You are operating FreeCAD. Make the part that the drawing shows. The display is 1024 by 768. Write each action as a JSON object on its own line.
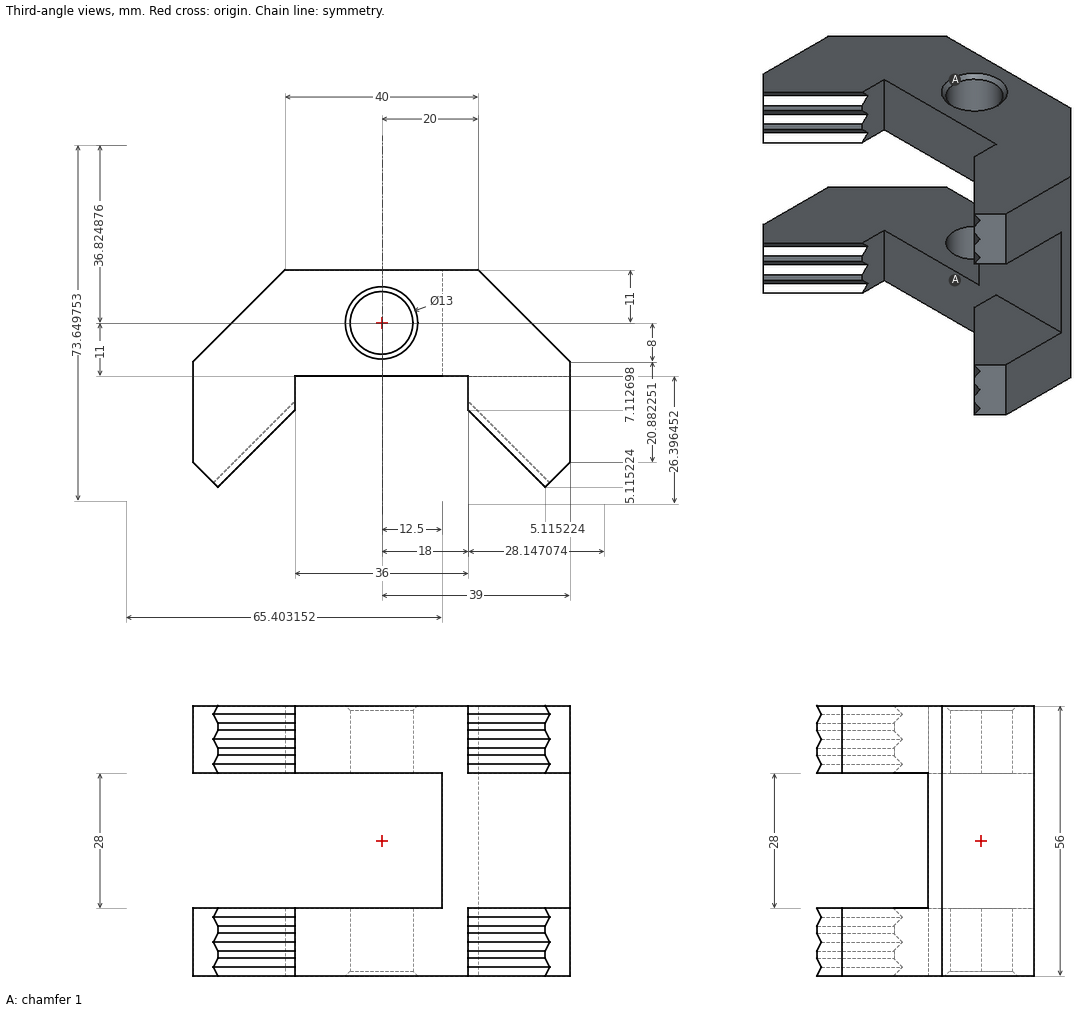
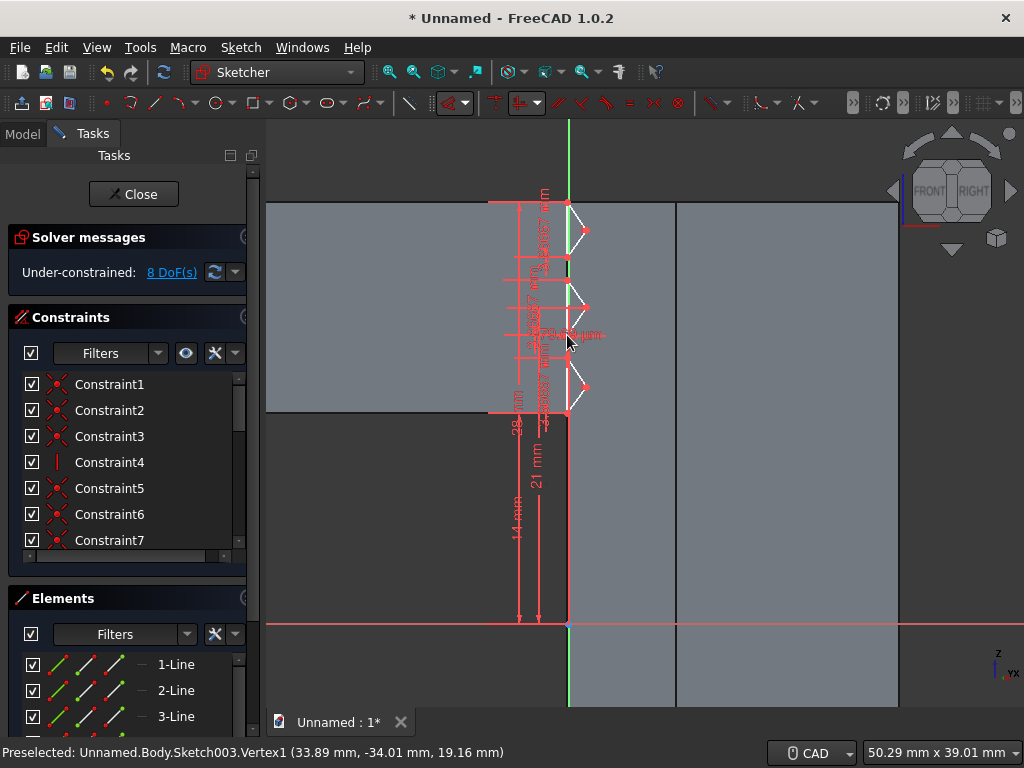
{"action": "scroll", "coordinate": [567, 413], "scroll_direction": "up", "scroll_amount": 18}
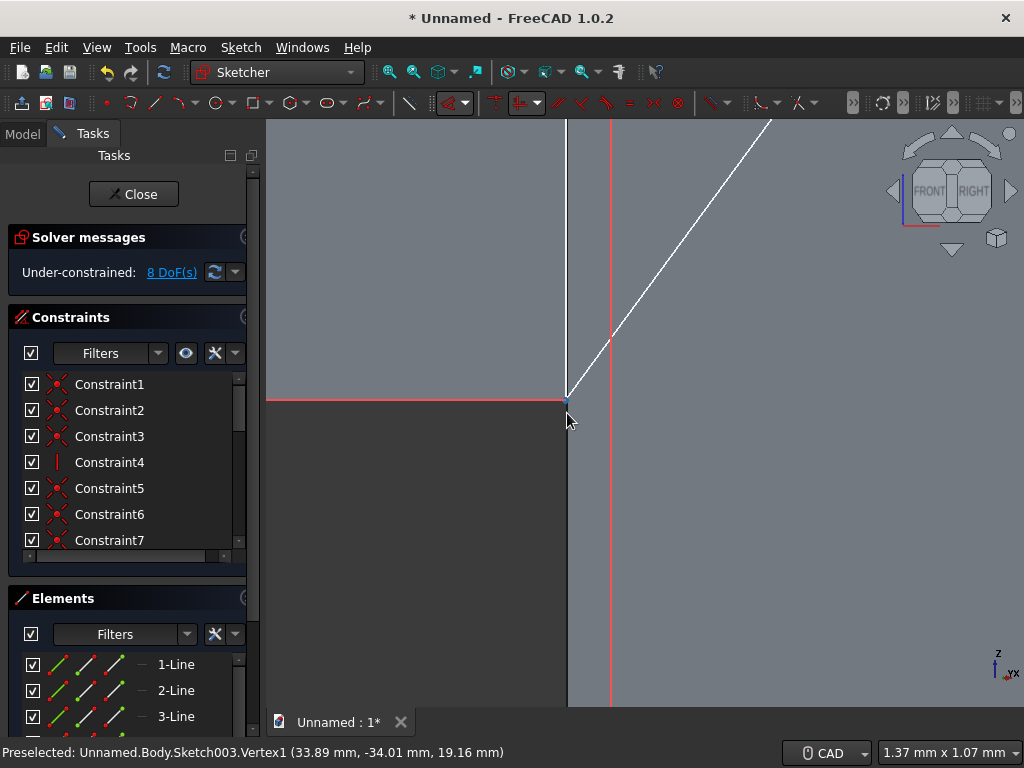
{"action": "left_click", "coordinate": [566, 400]}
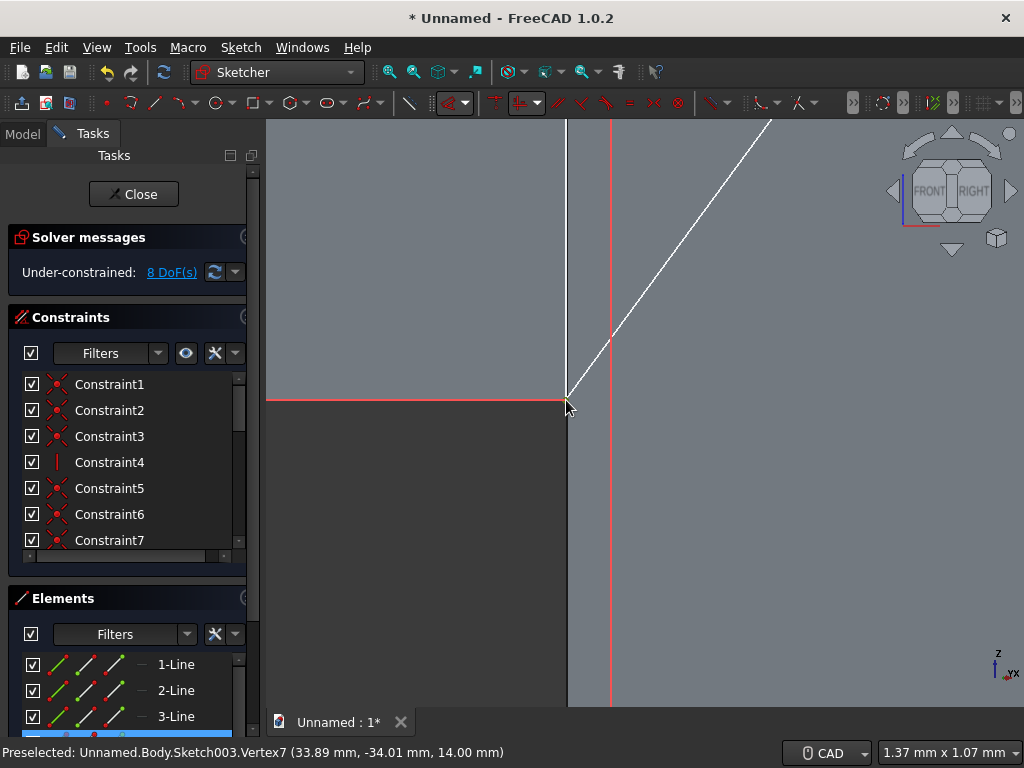
{"action": "key", "text": "l"}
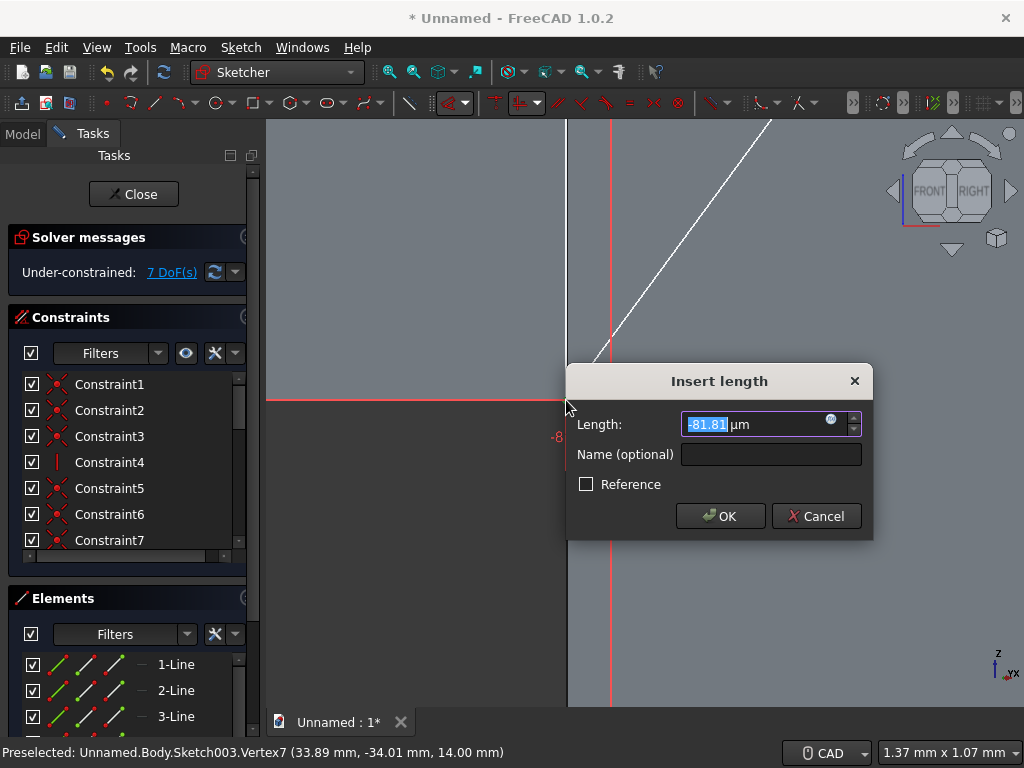
{"action": "key", "text": "ctrl+a"}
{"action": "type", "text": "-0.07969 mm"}
{"action": "key", "text": "Return"}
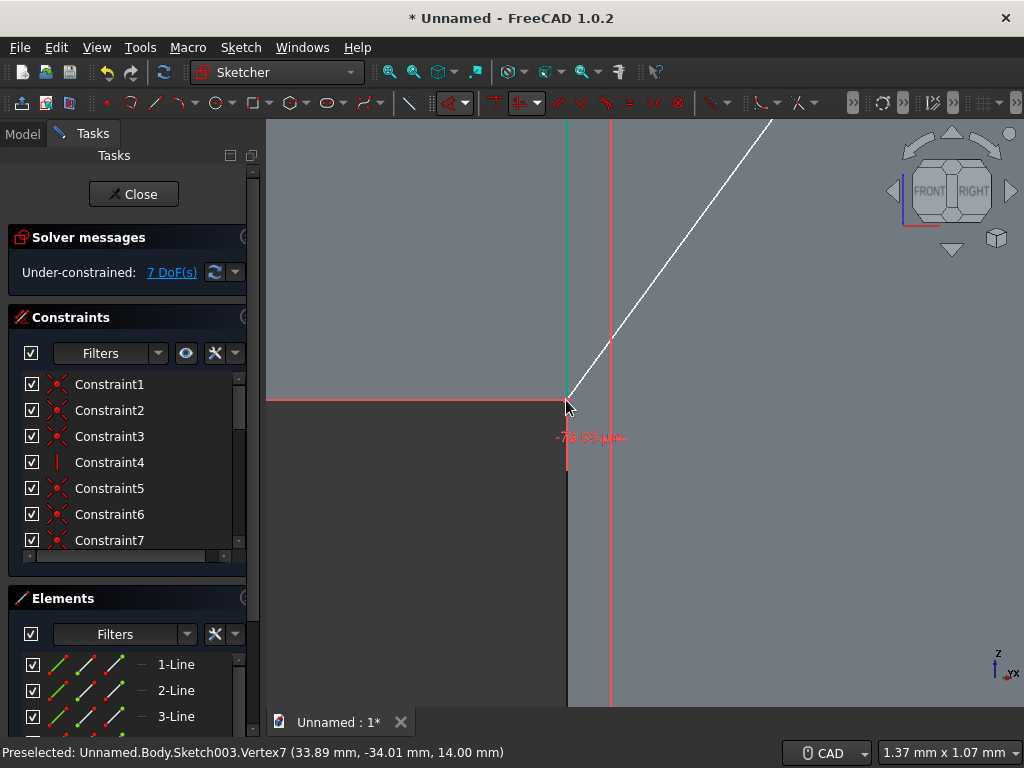
{"action": "scroll", "coordinate": [567, 413], "scroll_direction": "down", "scroll_amount": 18}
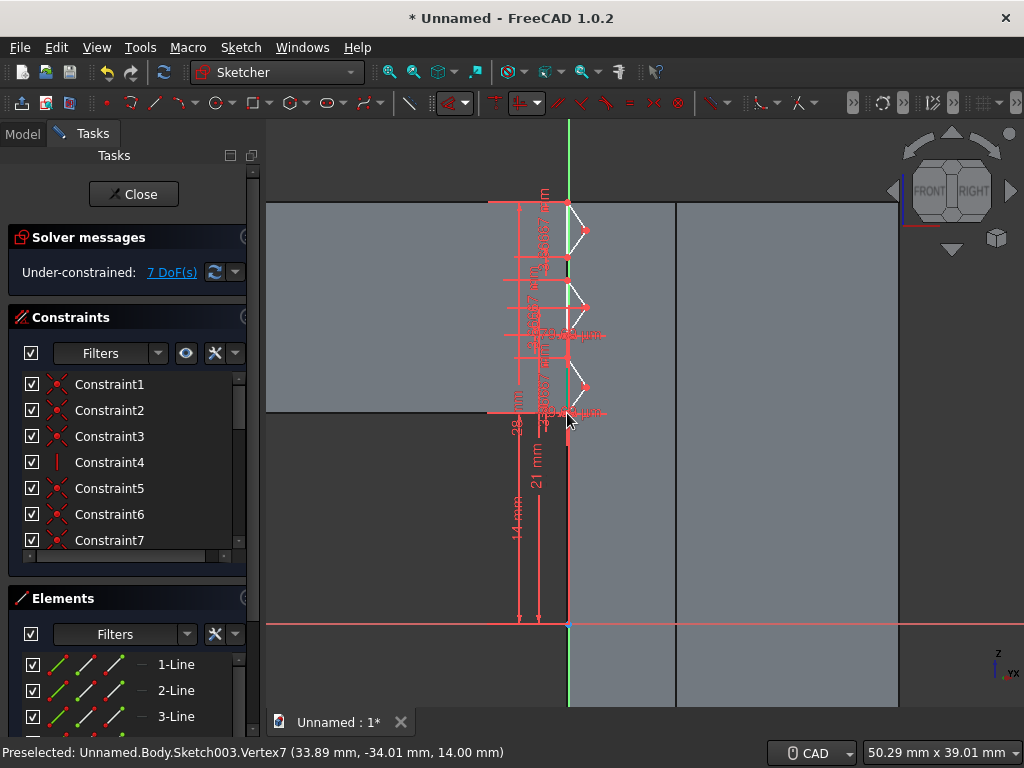
{"action": "scroll", "coordinate": [567, 257], "scroll_direction": "up", "scroll_amount": 18}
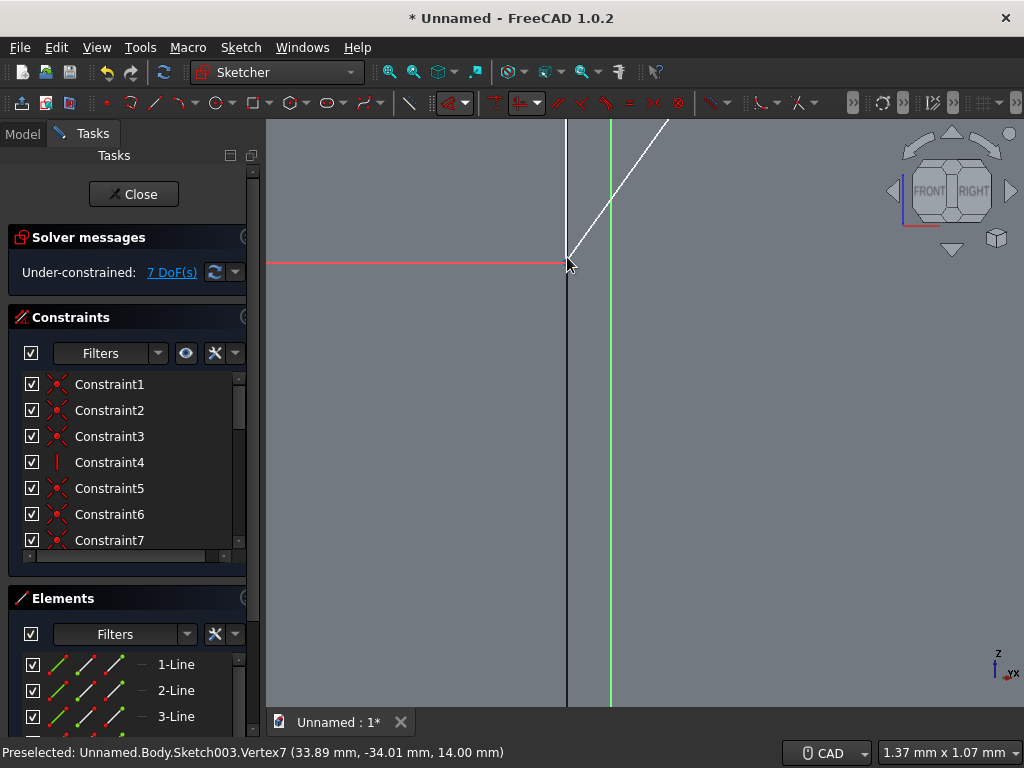
{"action": "left_click", "coordinate": [566, 263]}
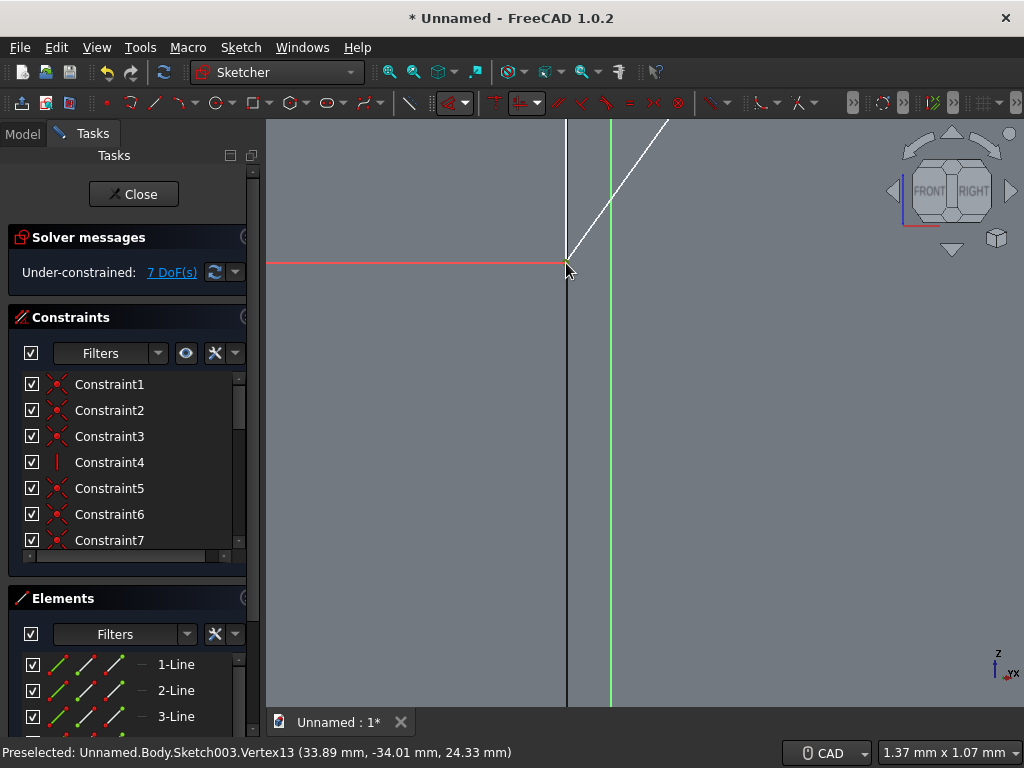
{"action": "key", "text": "l"}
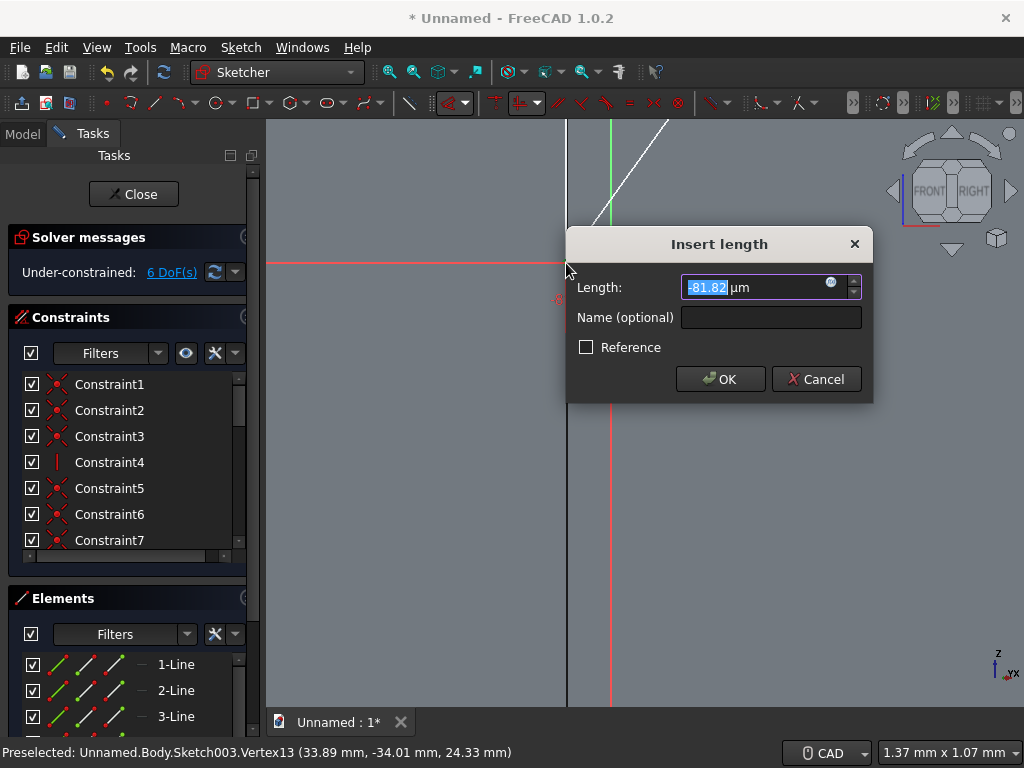
{"action": "key", "text": "ctrl+a"}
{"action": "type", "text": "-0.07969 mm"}
{"action": "key", "text": "Return"}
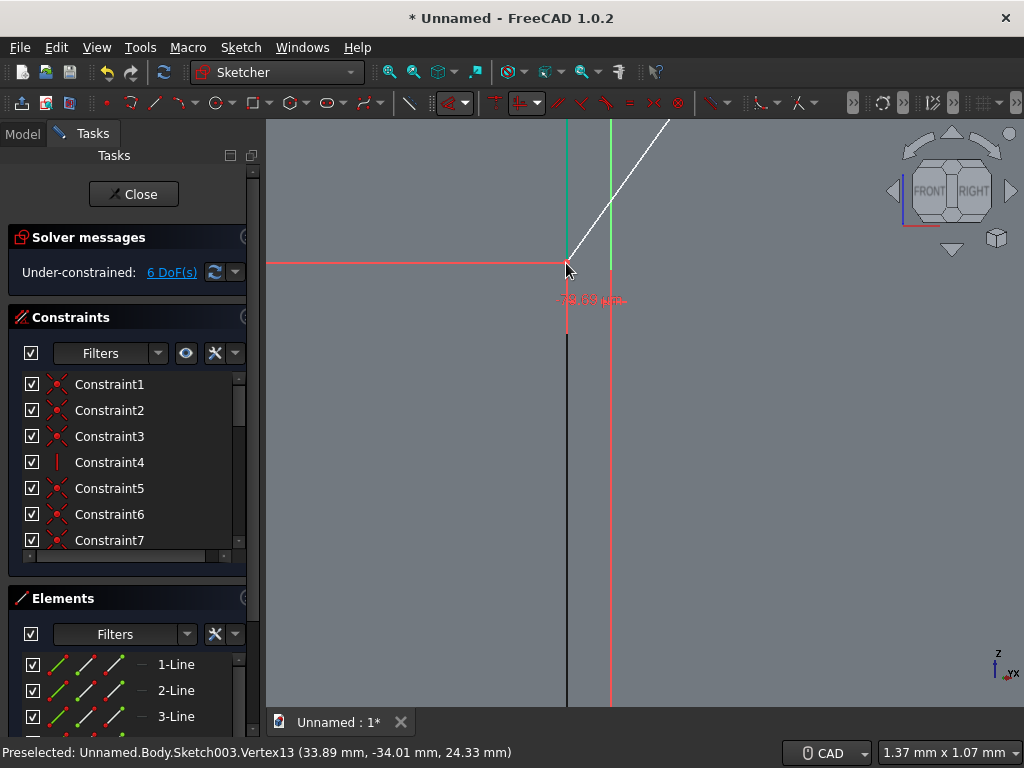
{"action": "scroll", "coordinate": [567, 257], "scroll_direction": "down", "scroll_amount": 18}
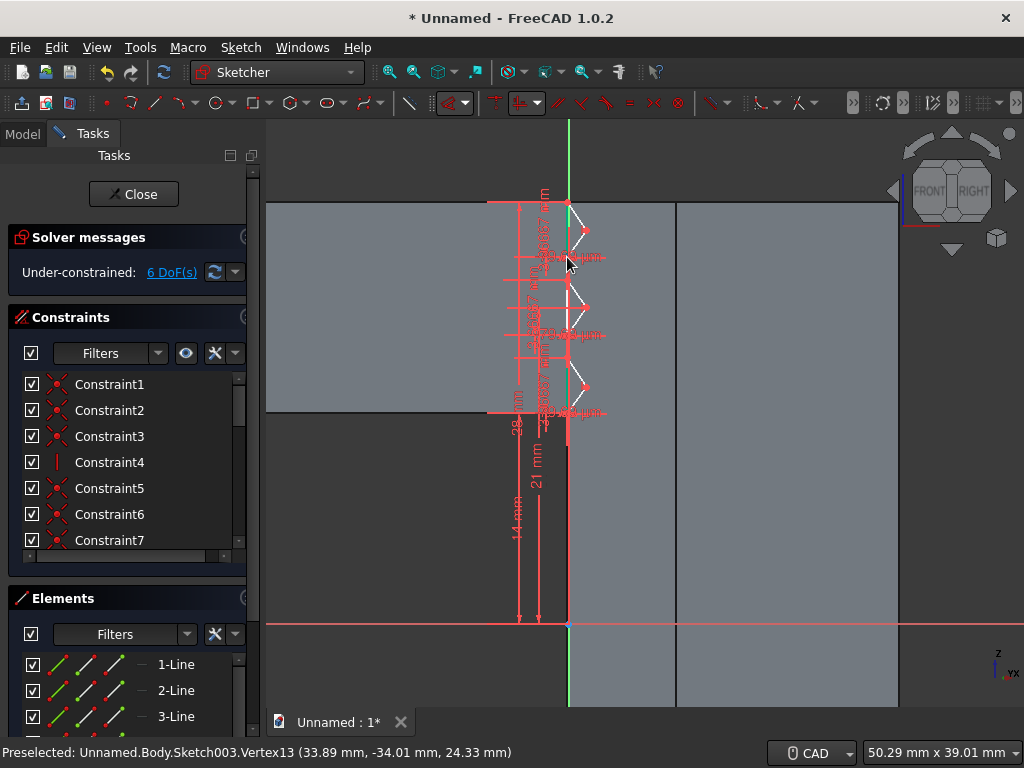
{"action": "scroll", "coordinate": [587, 308], "scroll_direction": "up", "scroll_amount": 4}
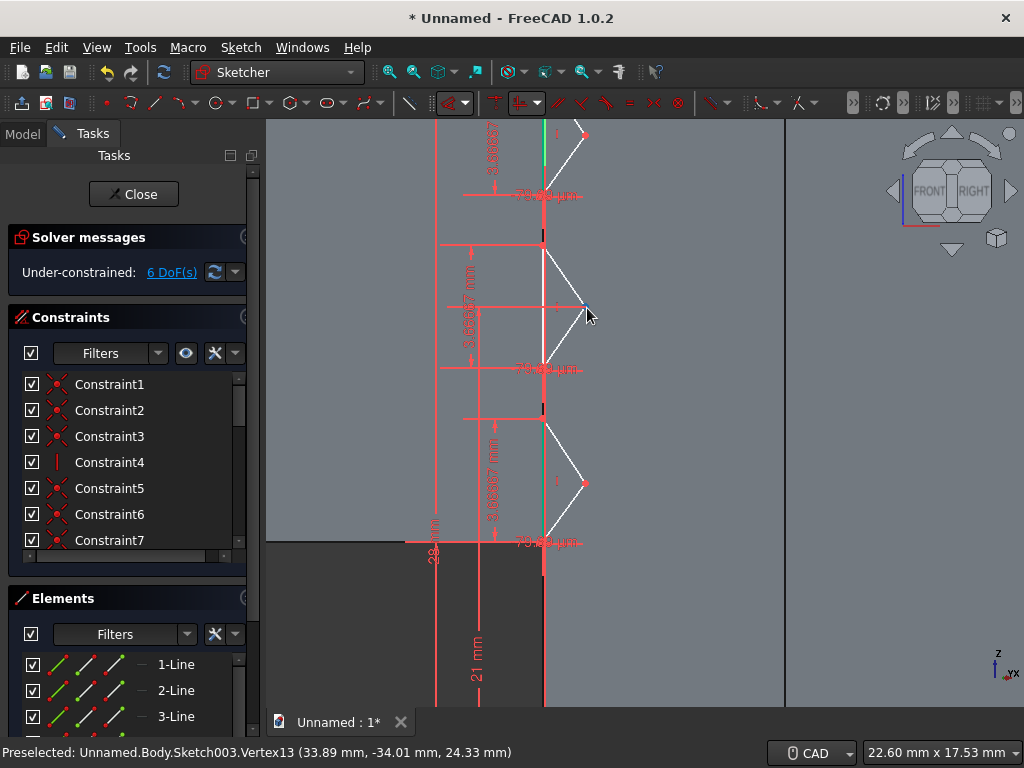
{"action": "left_click", "coordinate": [585, 307]}